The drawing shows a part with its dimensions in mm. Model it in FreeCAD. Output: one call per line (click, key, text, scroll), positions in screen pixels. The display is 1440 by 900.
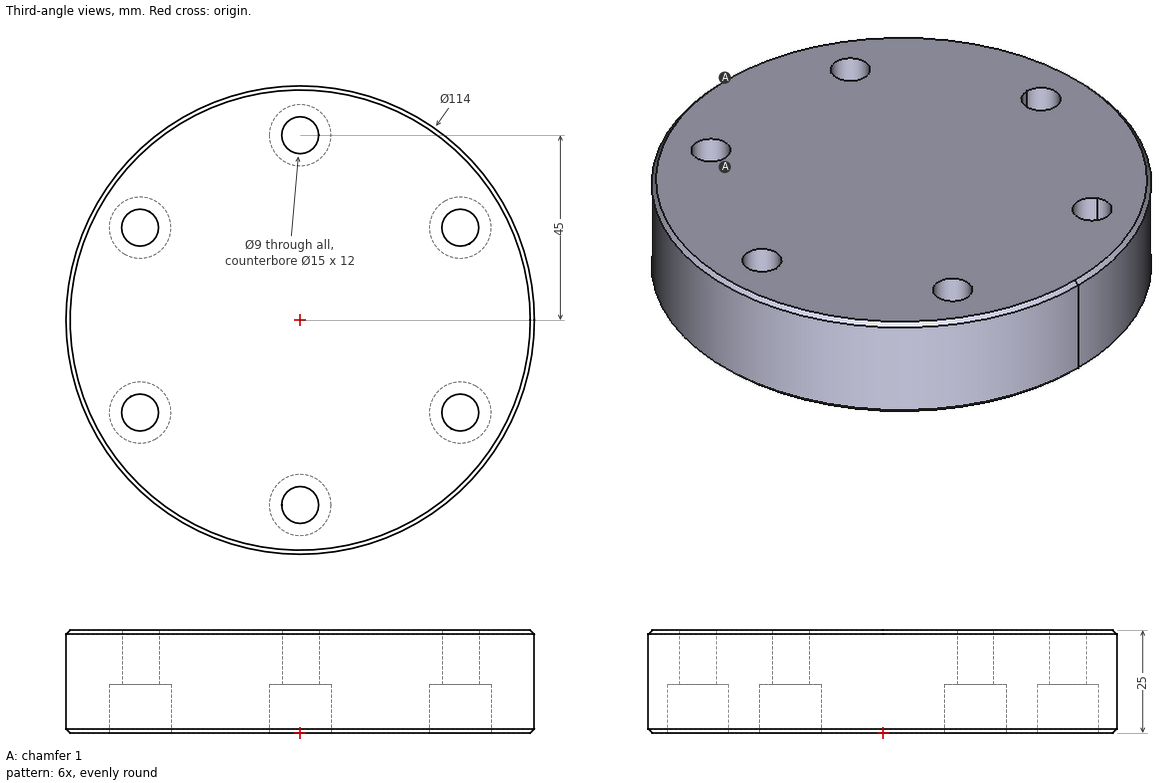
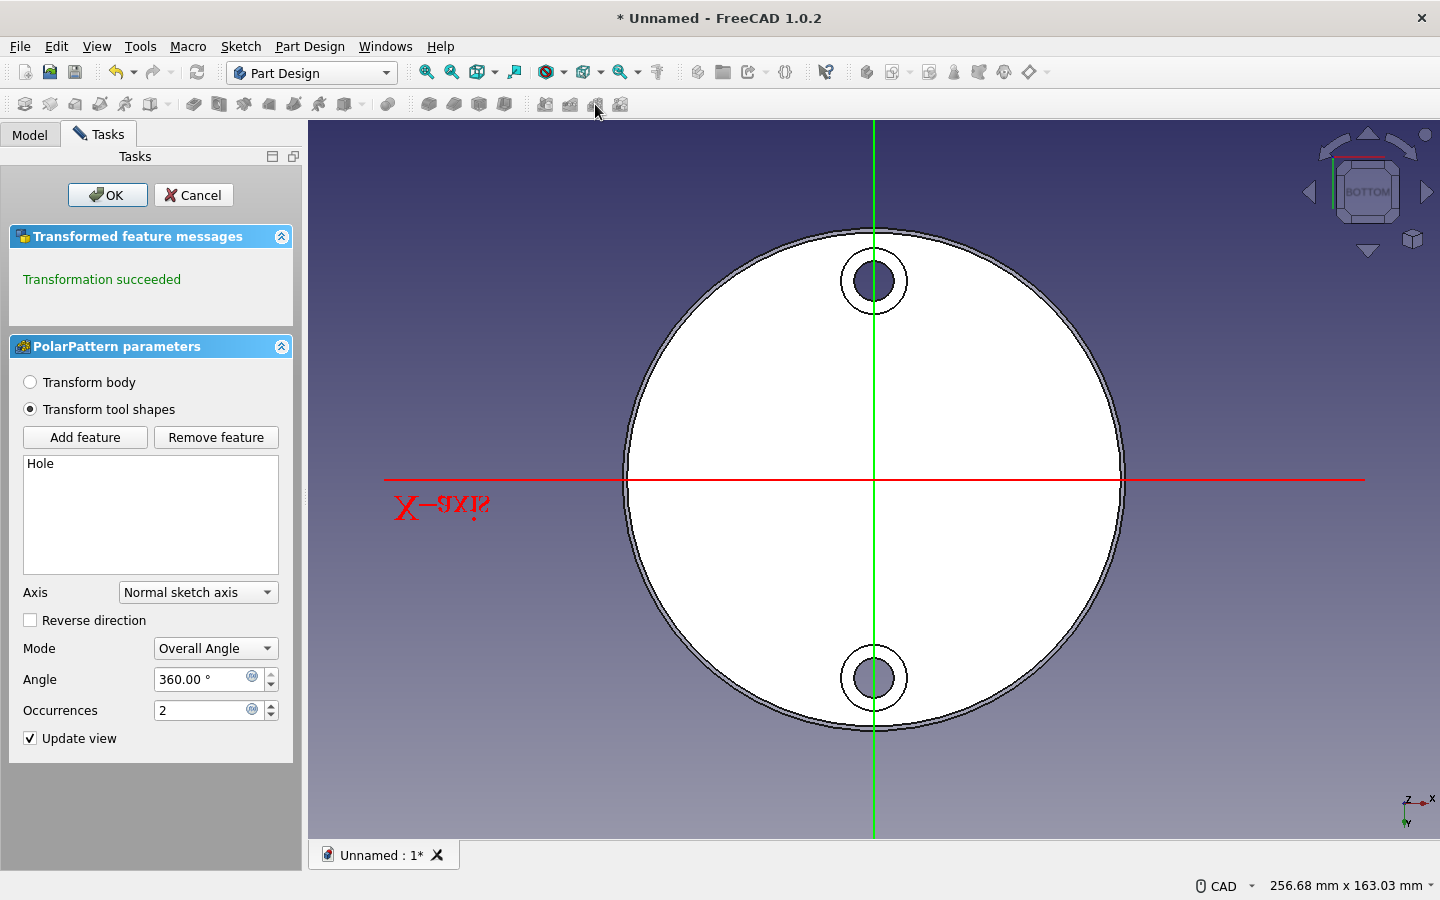
click(199, 592)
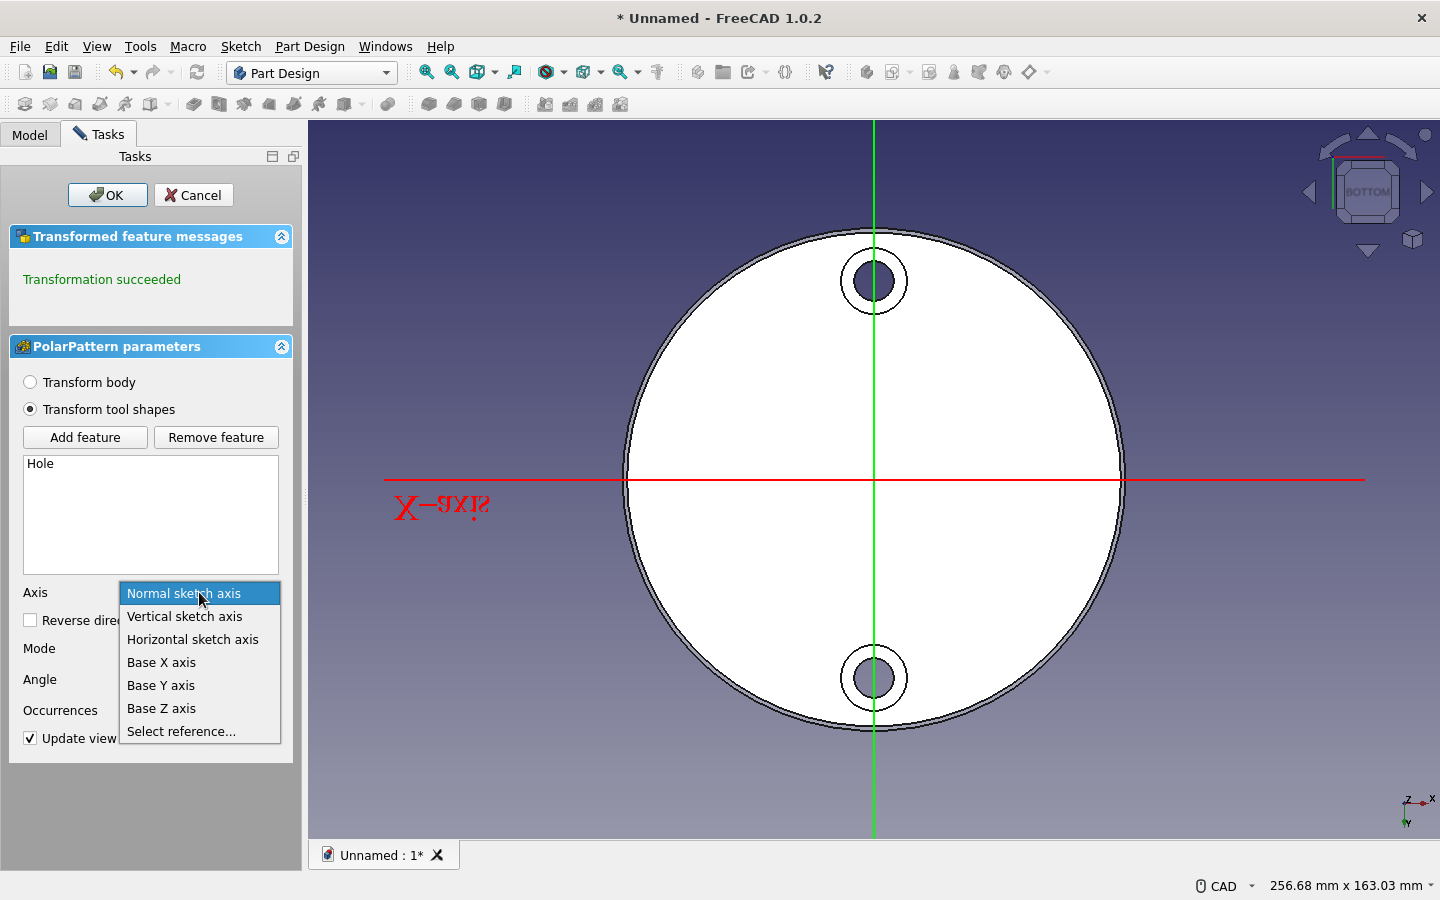
click(198, 708)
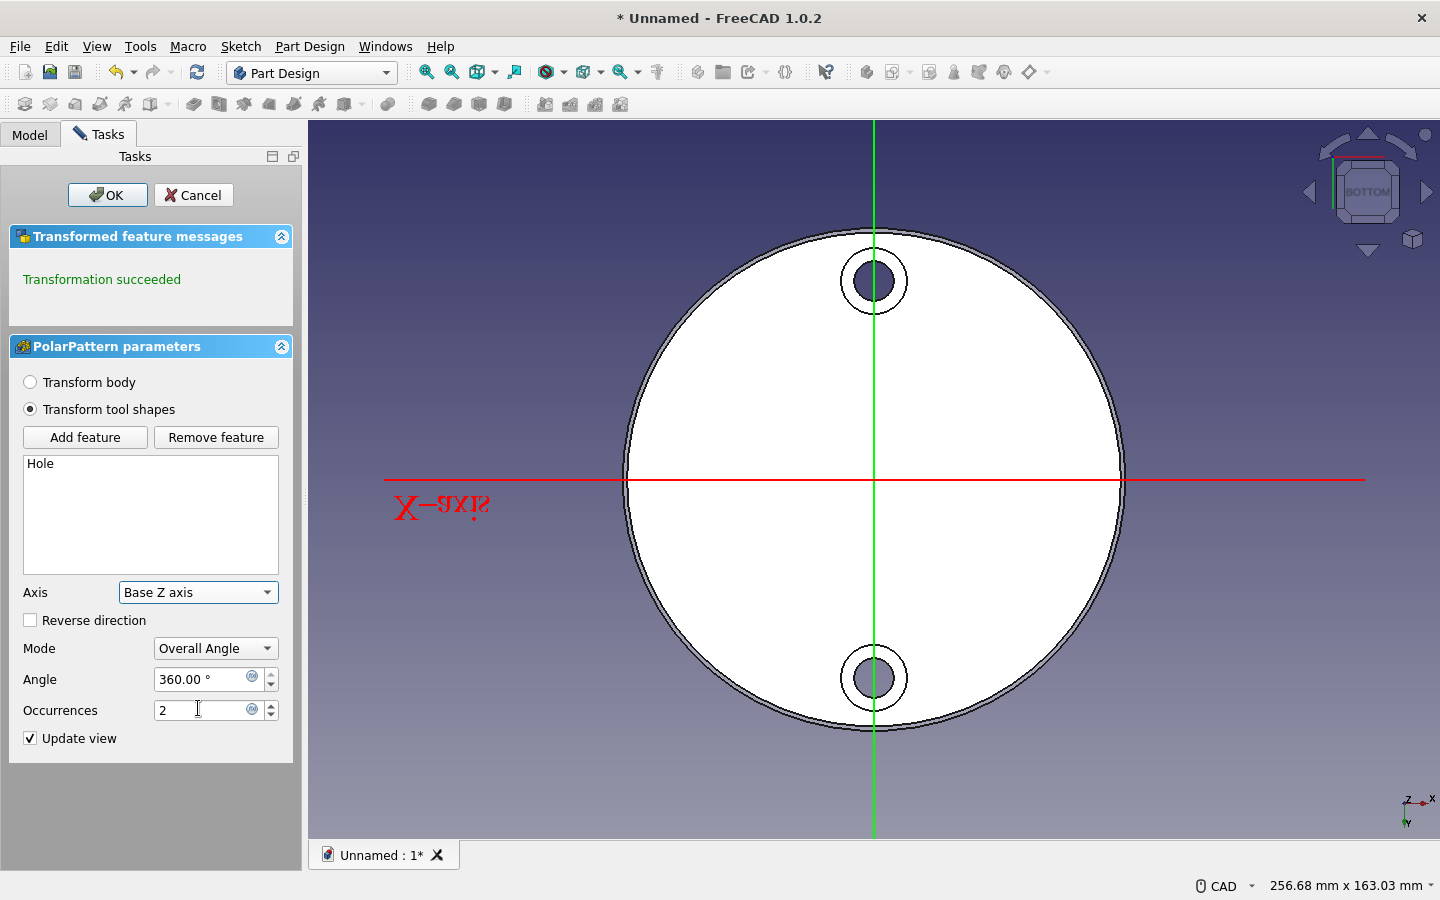
triple_click(210, 710)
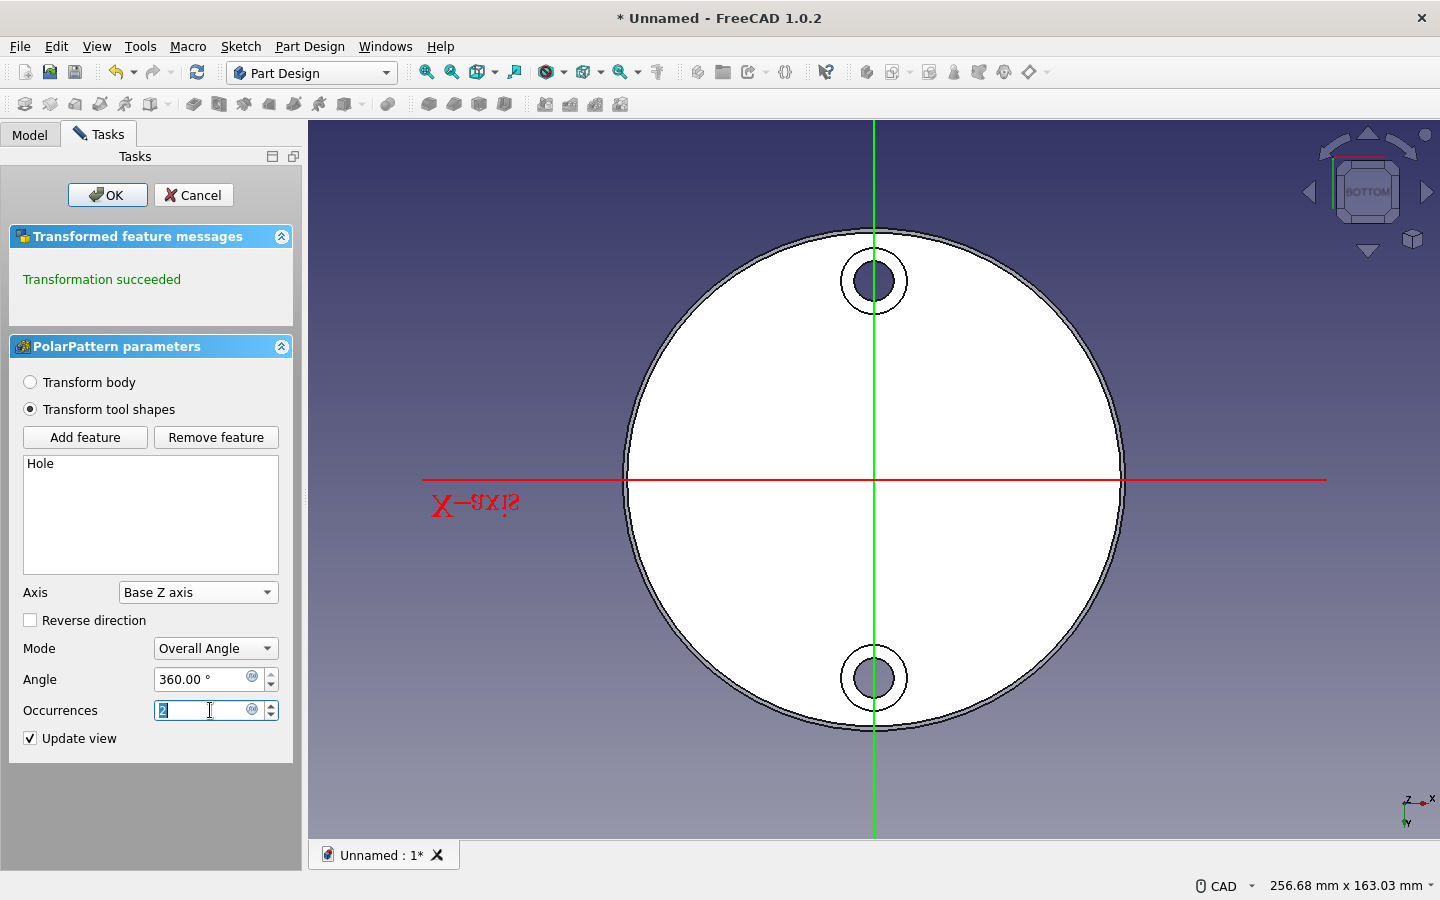
text(6)
key(Tab)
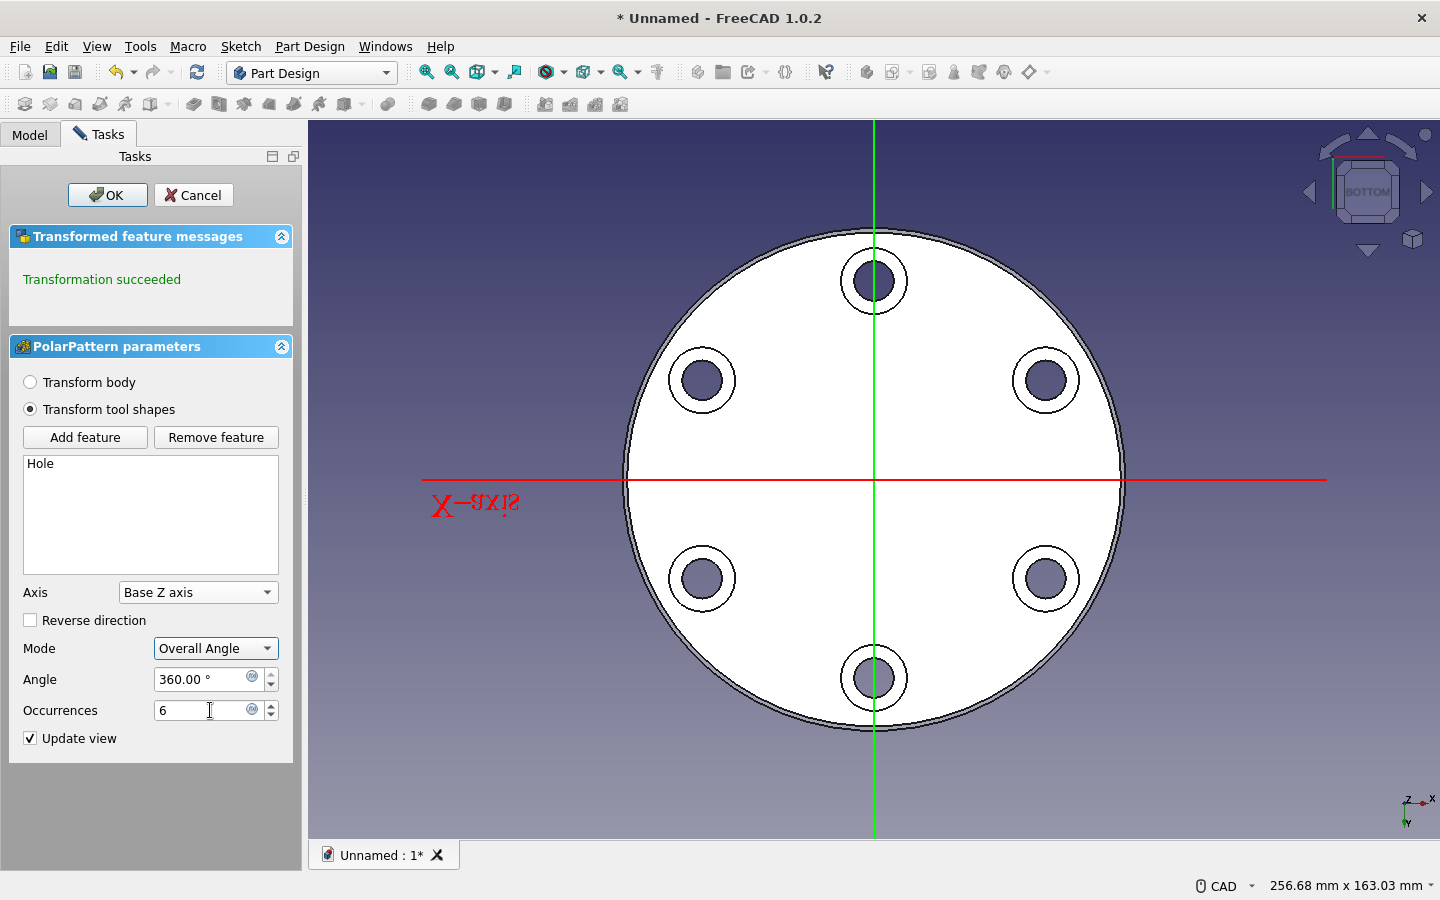
click(108, 195)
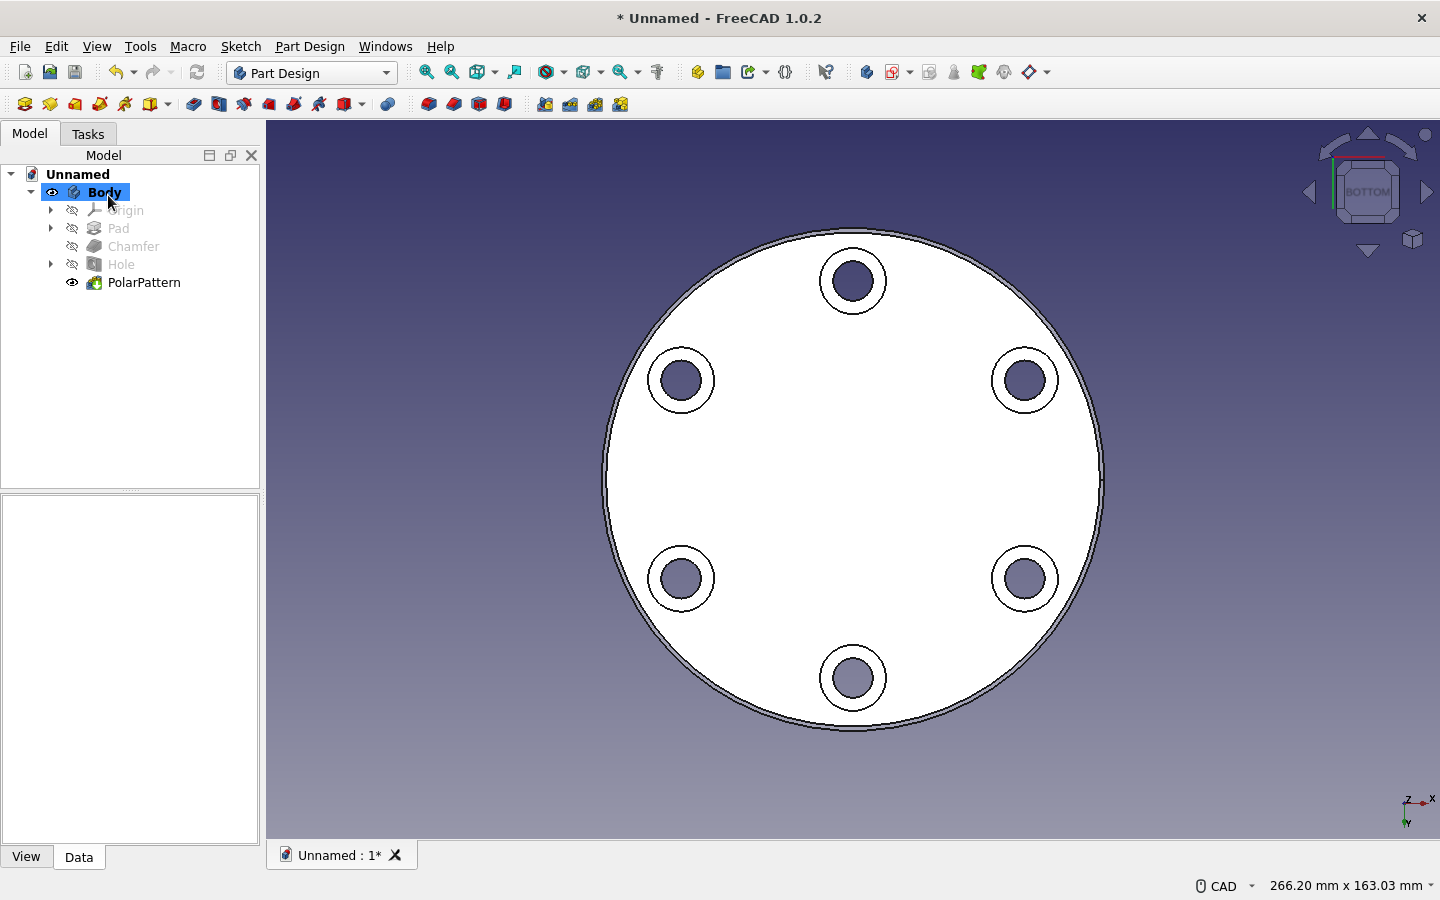
key(0)